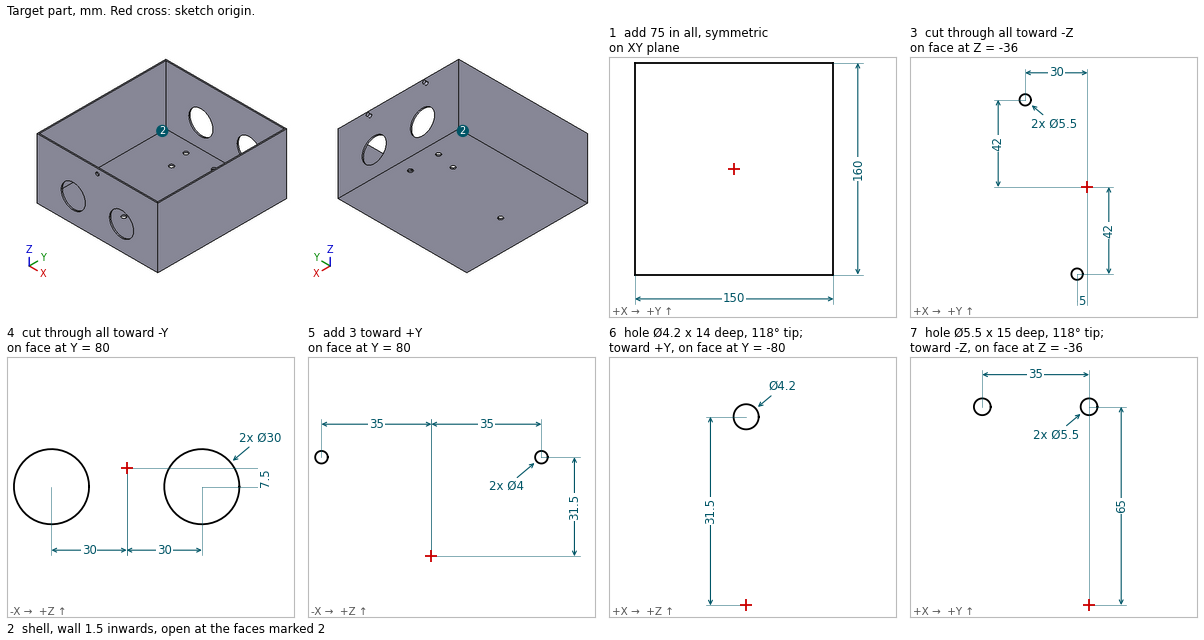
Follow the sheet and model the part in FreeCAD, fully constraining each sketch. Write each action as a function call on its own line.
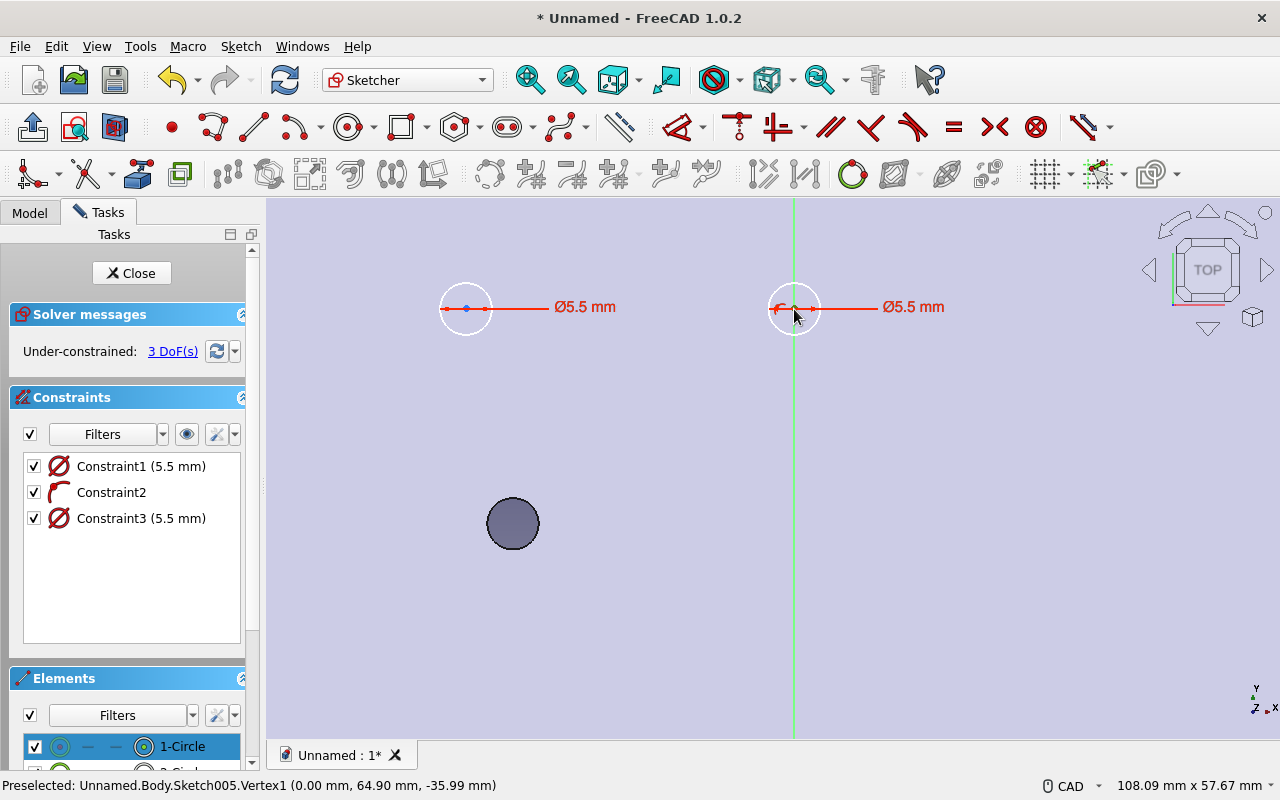
click(466, 309)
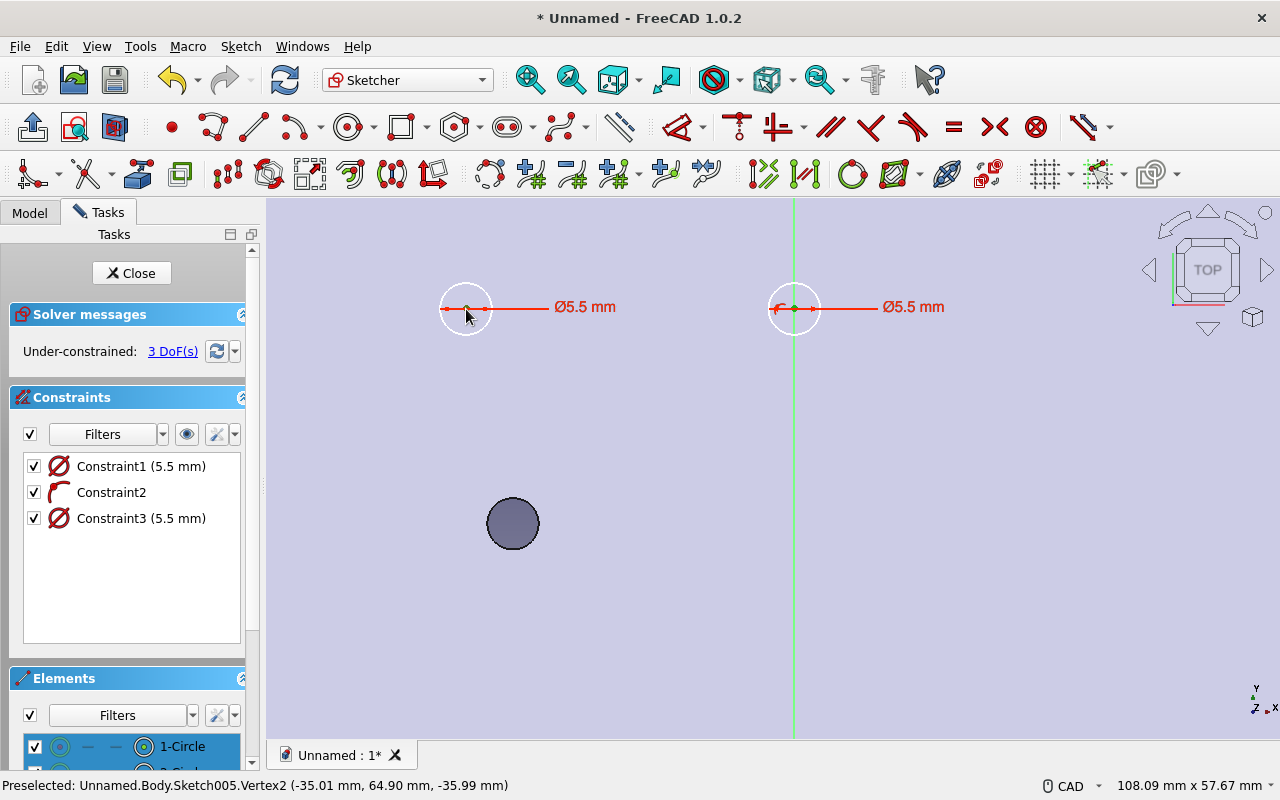
key(h)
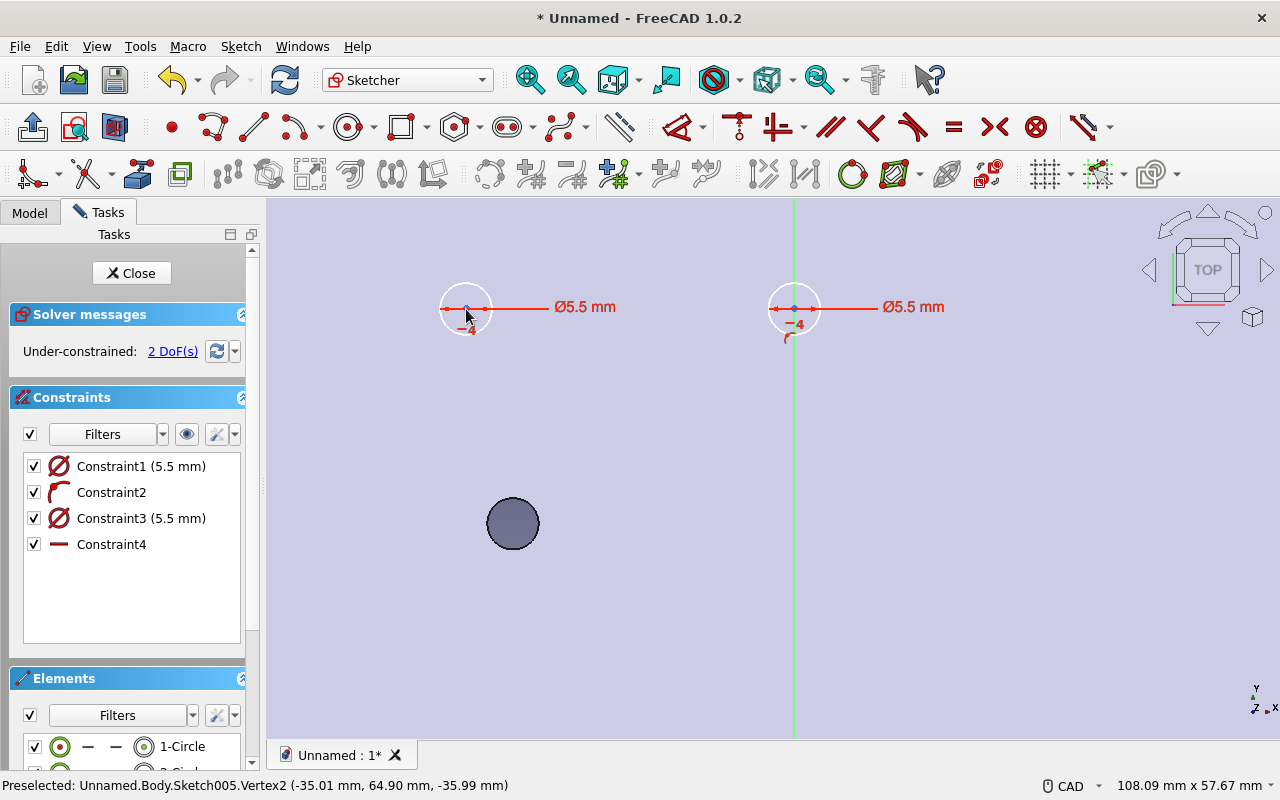
key(d)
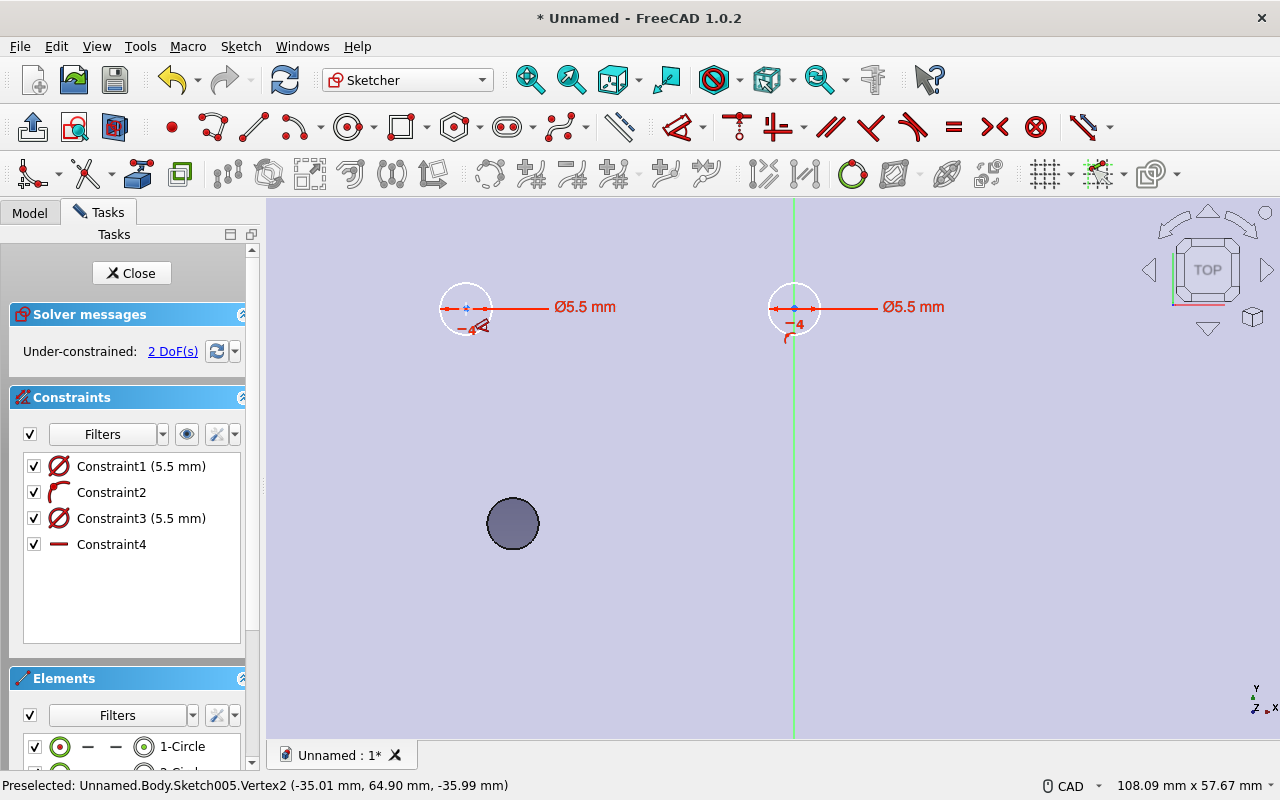
click(794, 309)
click(828, 510)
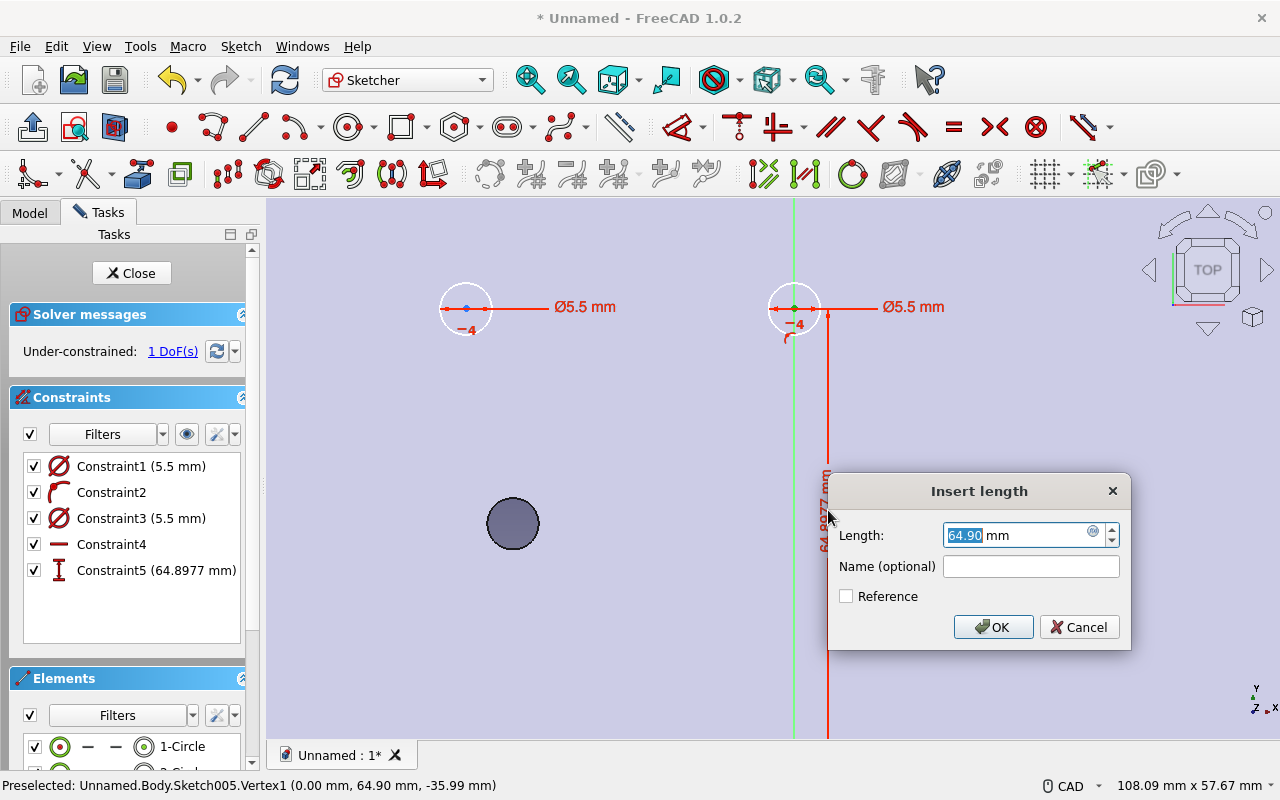
text(65)
key(Return)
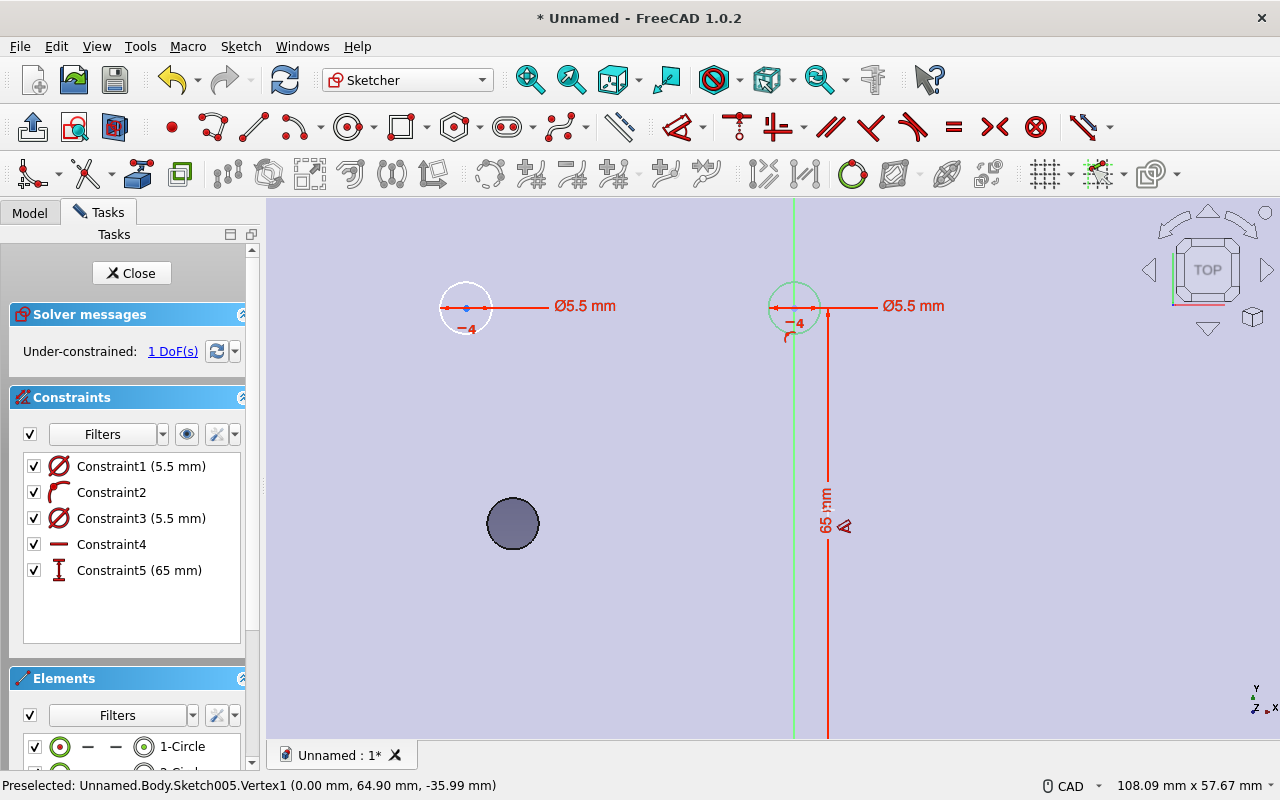
click(466, 308)
click(630, 274)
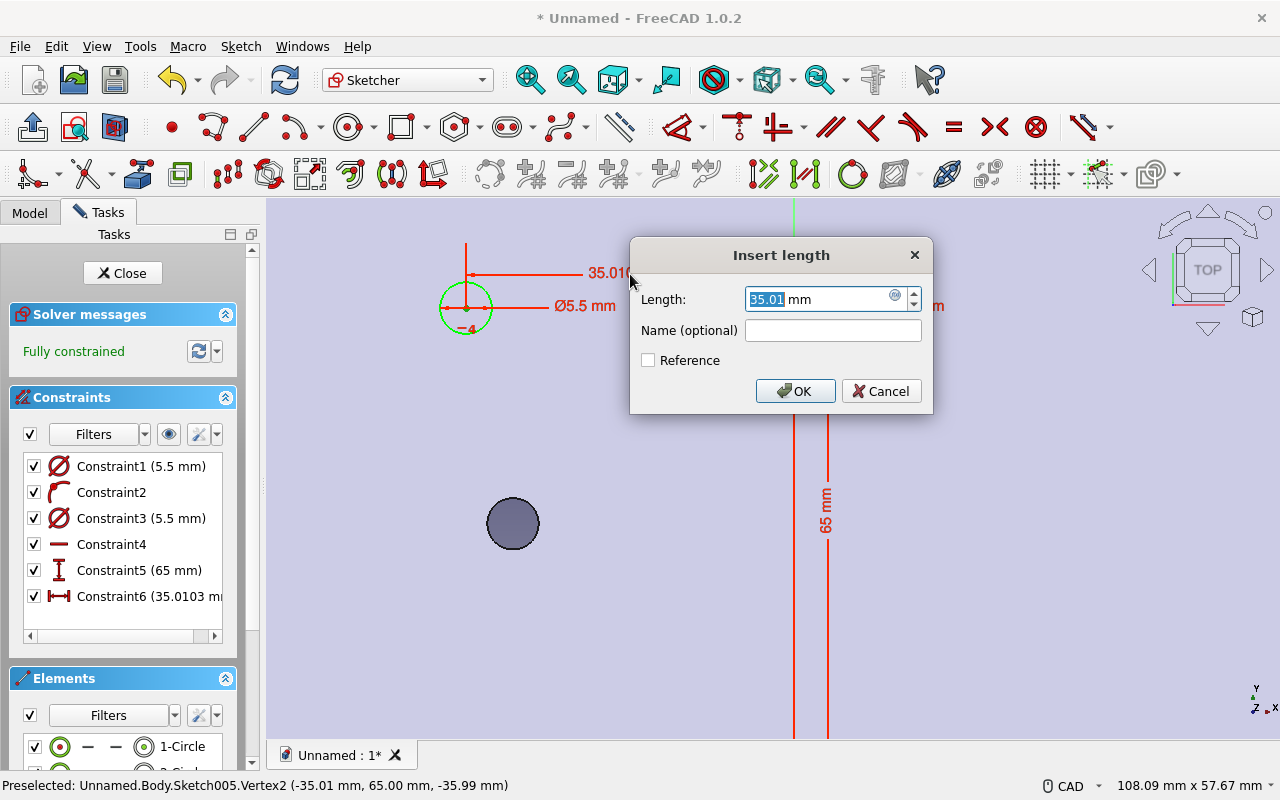
text(35)
key(Return)
key(Escape)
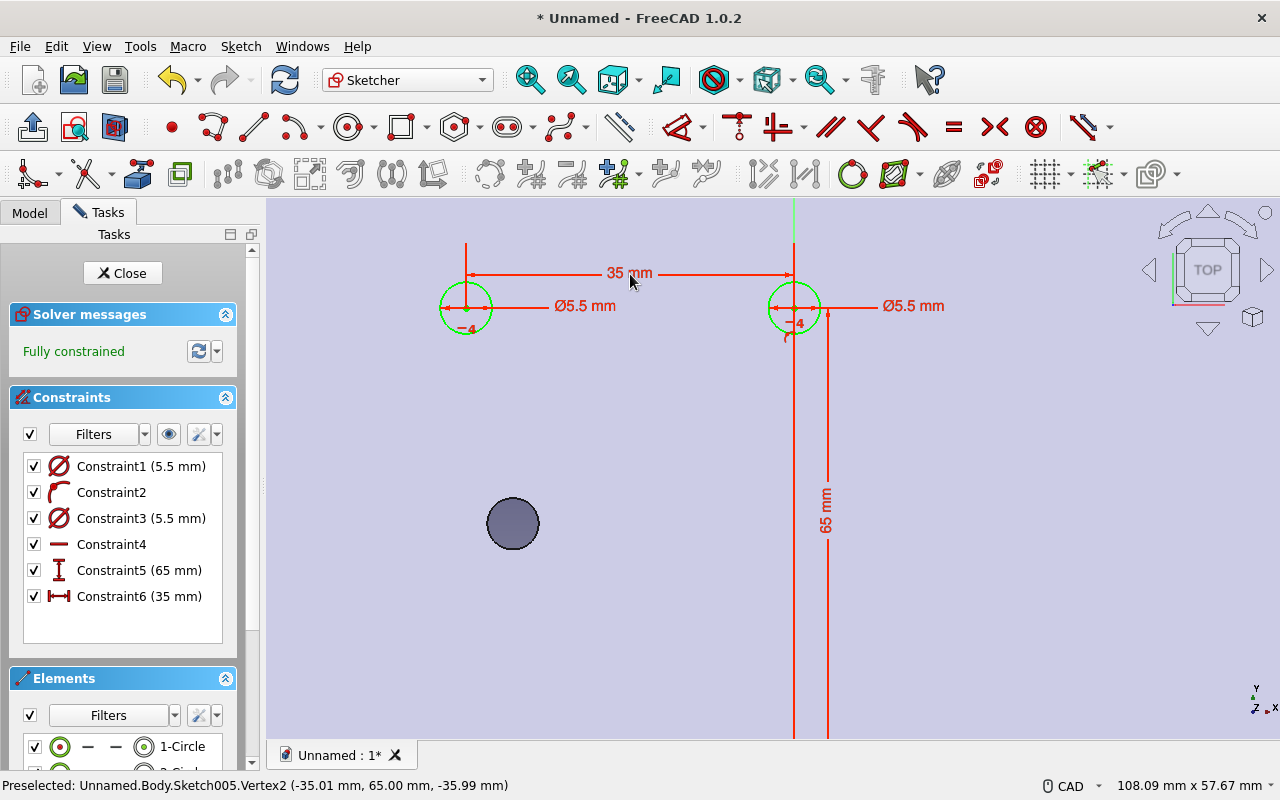
click(123, 273)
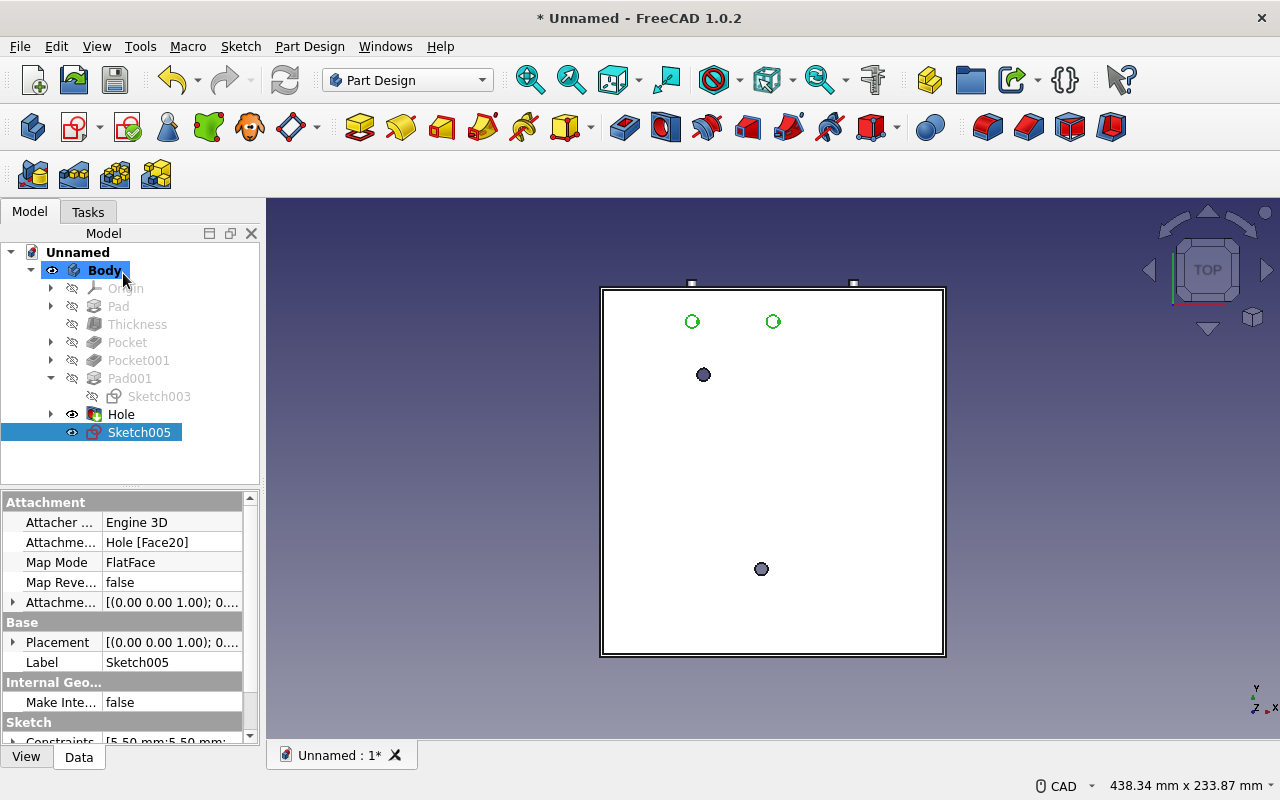
click(666, 128)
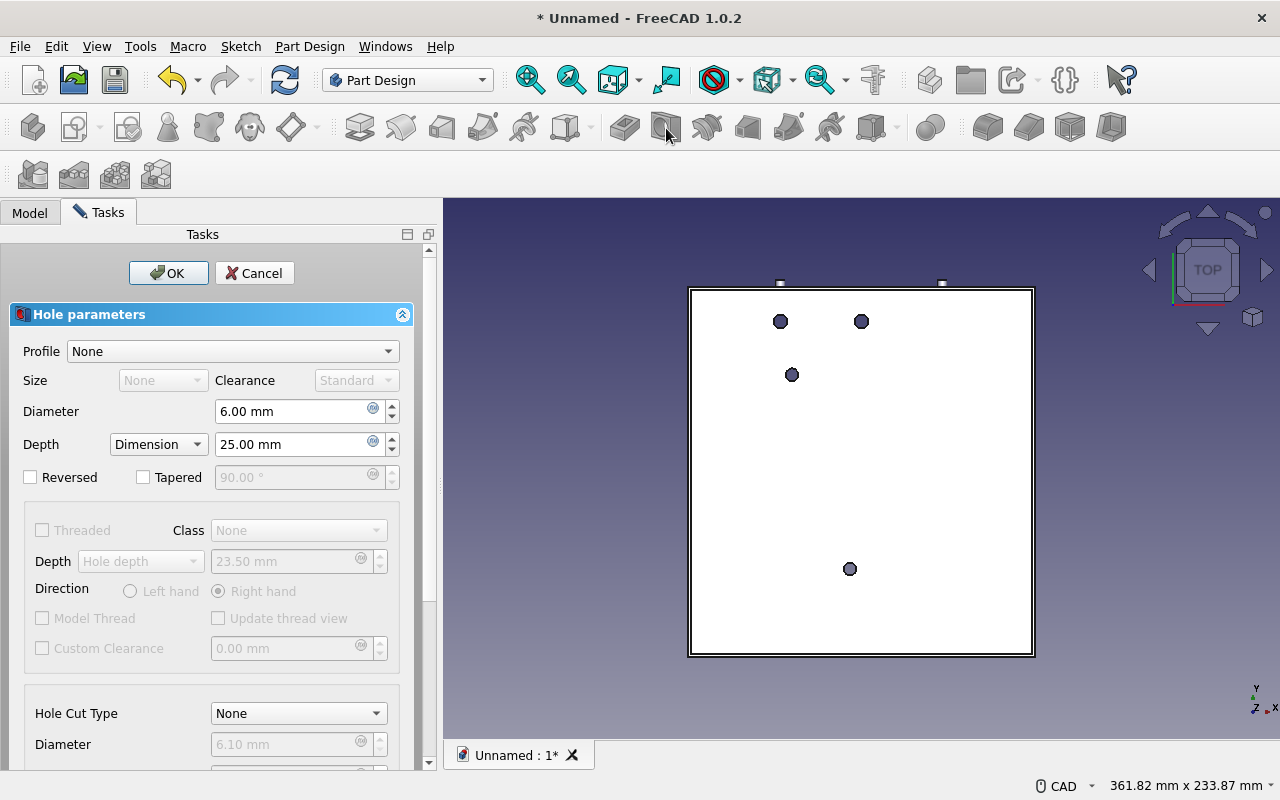
triple_click(300, 412)